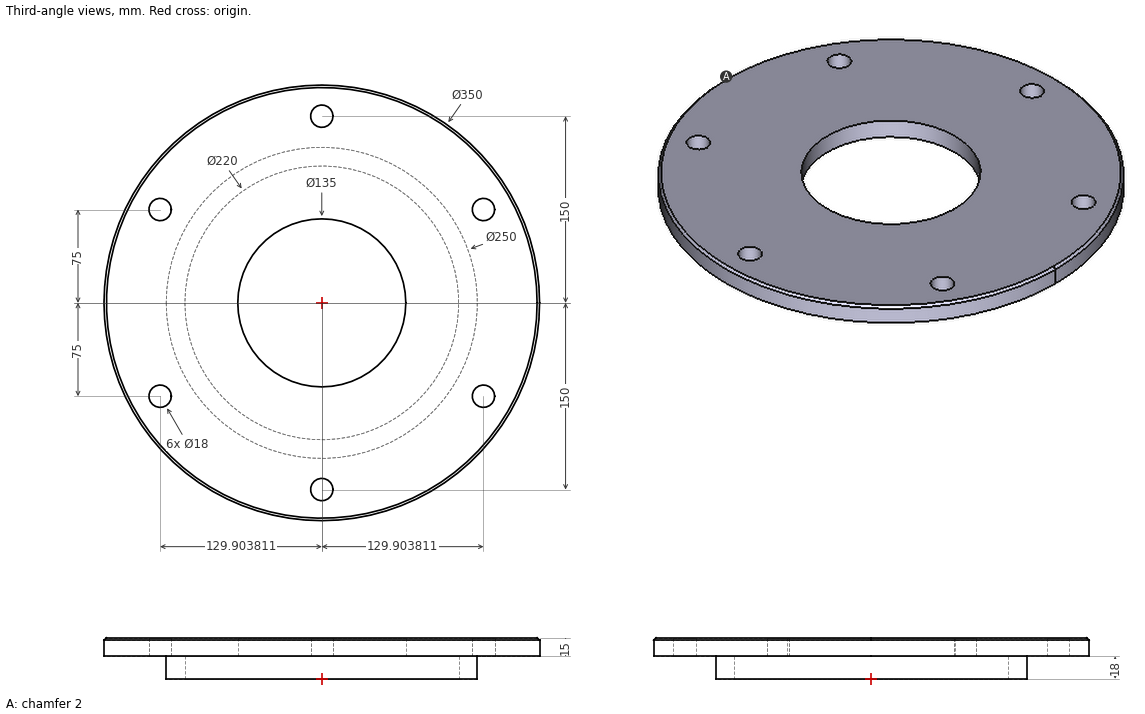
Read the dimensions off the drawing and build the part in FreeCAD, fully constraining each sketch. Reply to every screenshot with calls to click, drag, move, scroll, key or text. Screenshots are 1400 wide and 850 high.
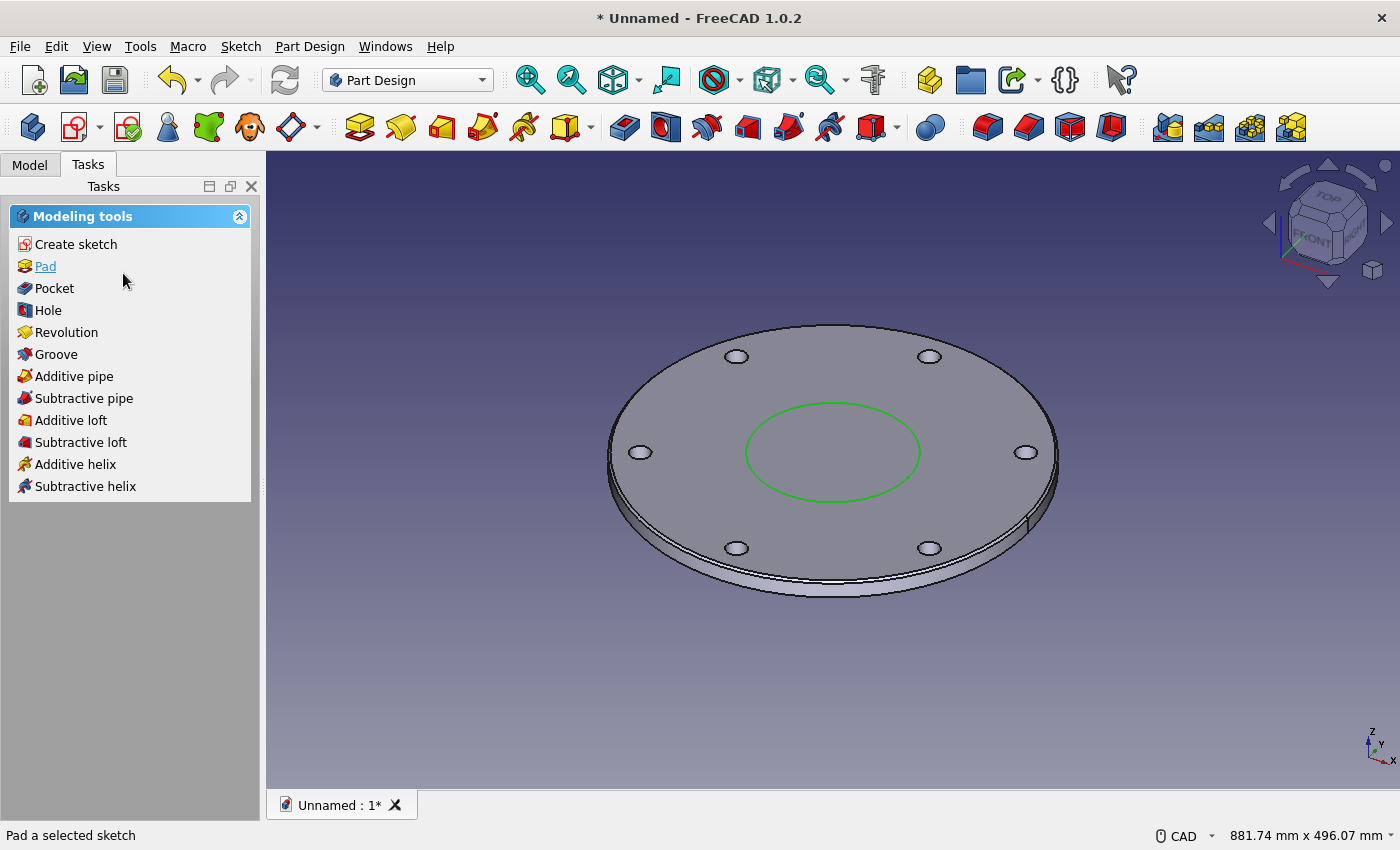
click(625, 128)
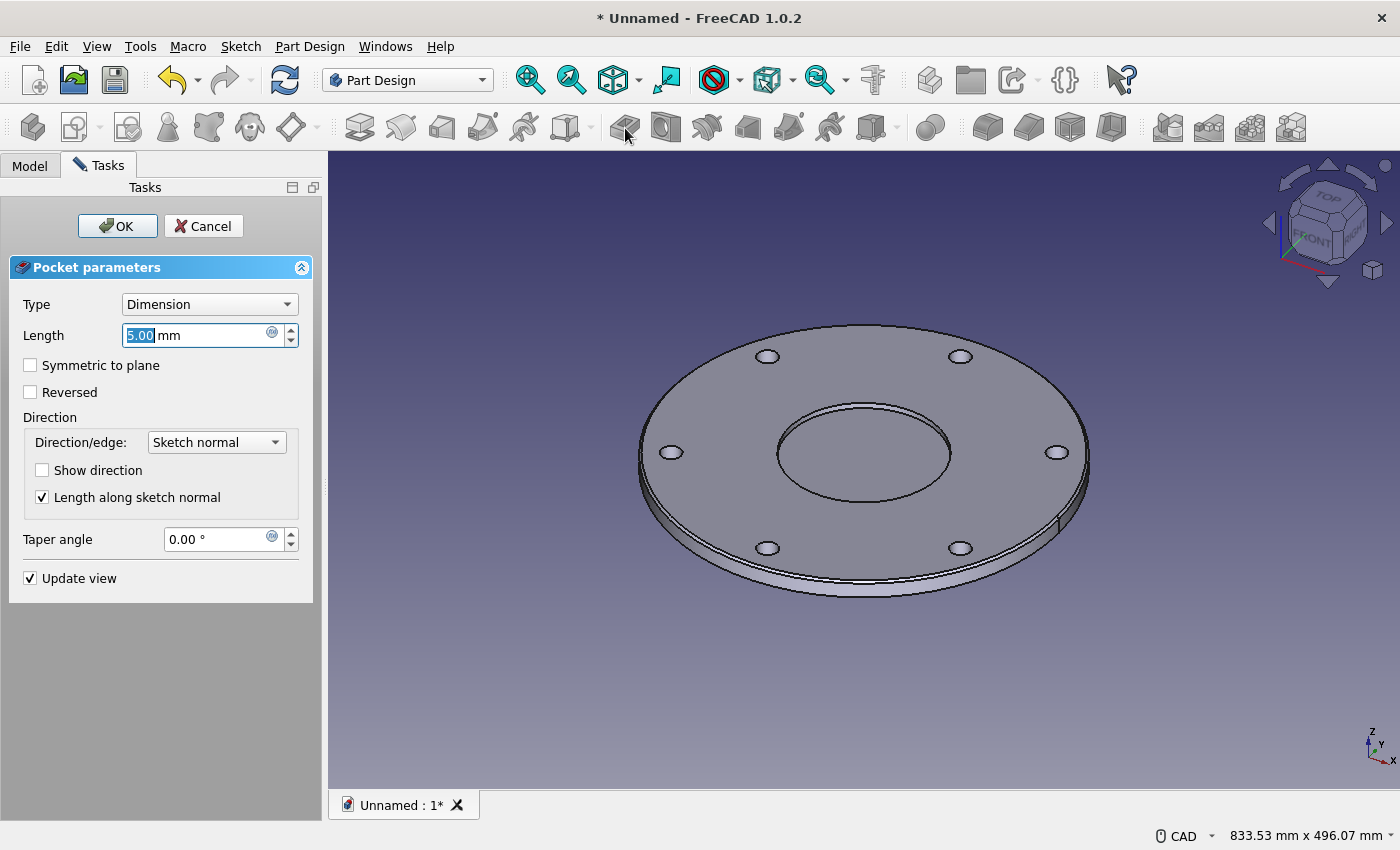
click(210, 304)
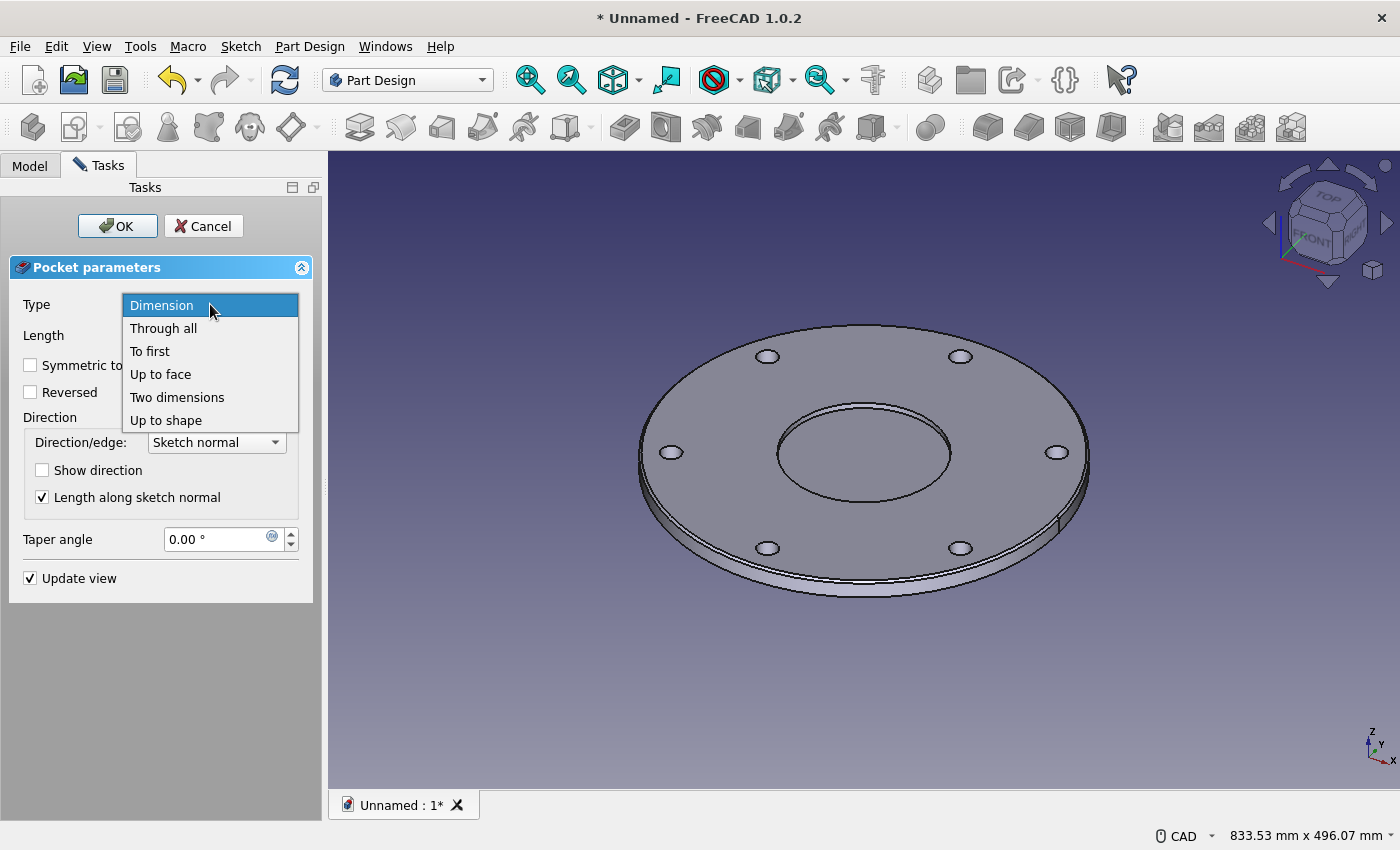
click(208, 328)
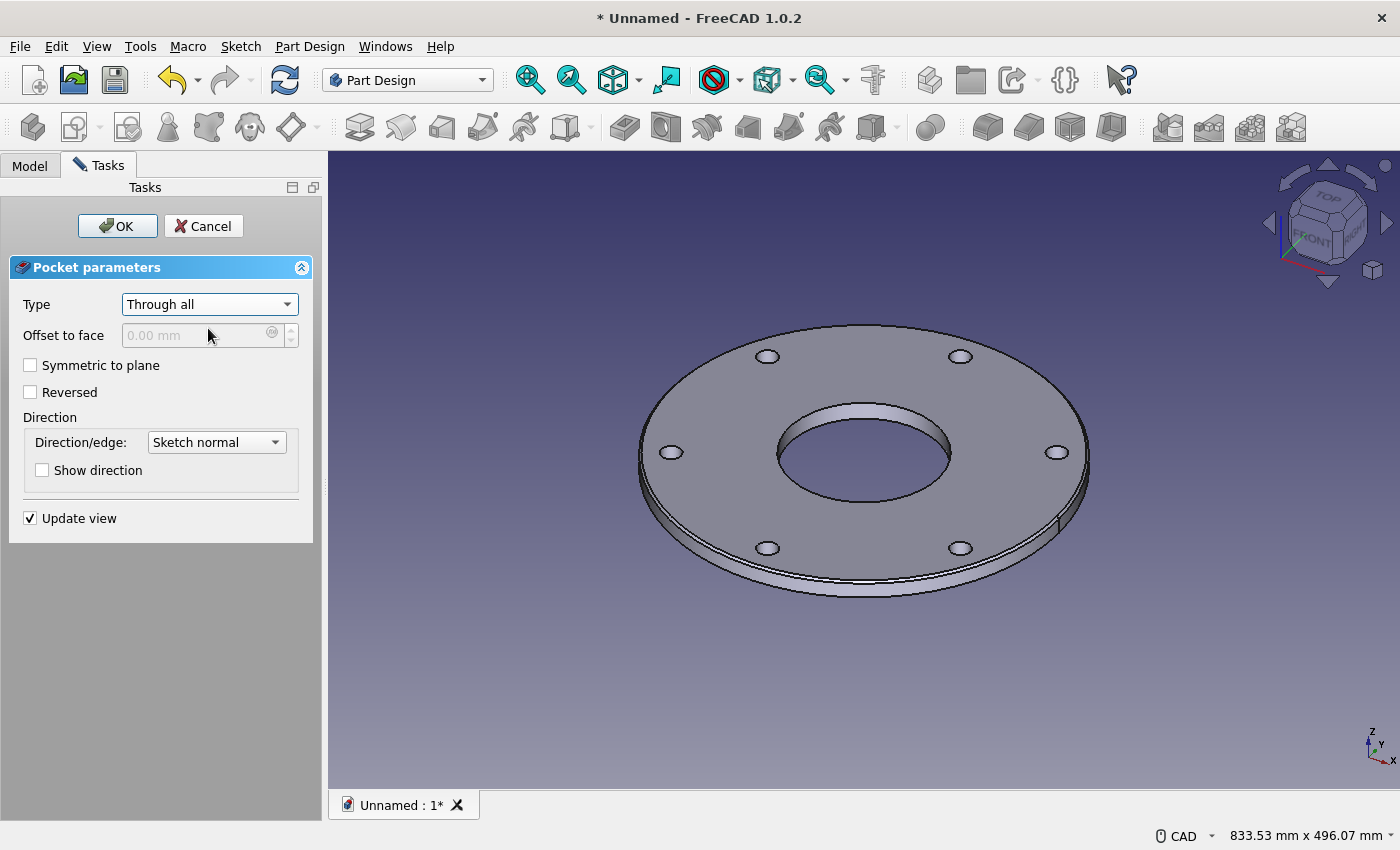
click(118, 226)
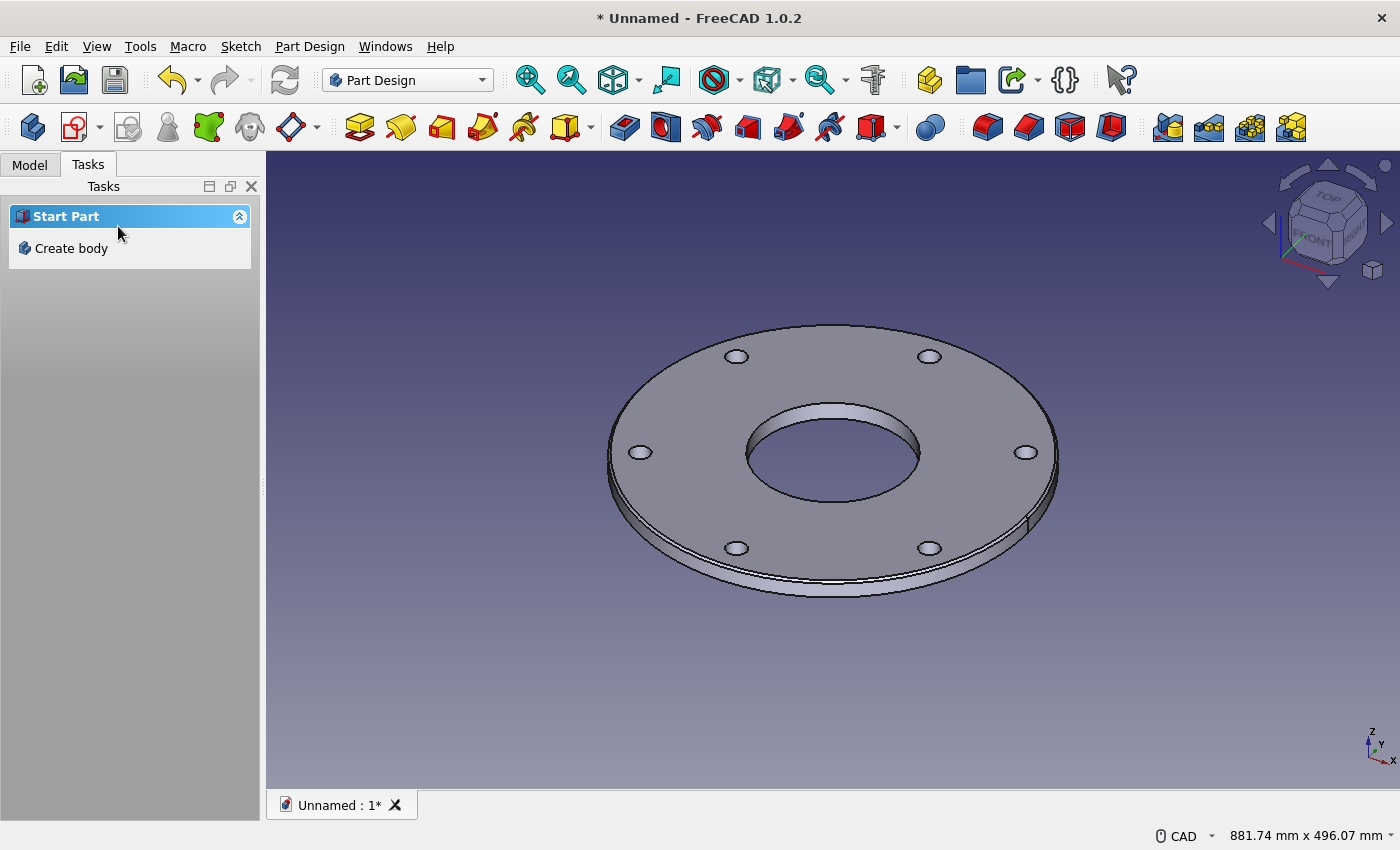
key(0)